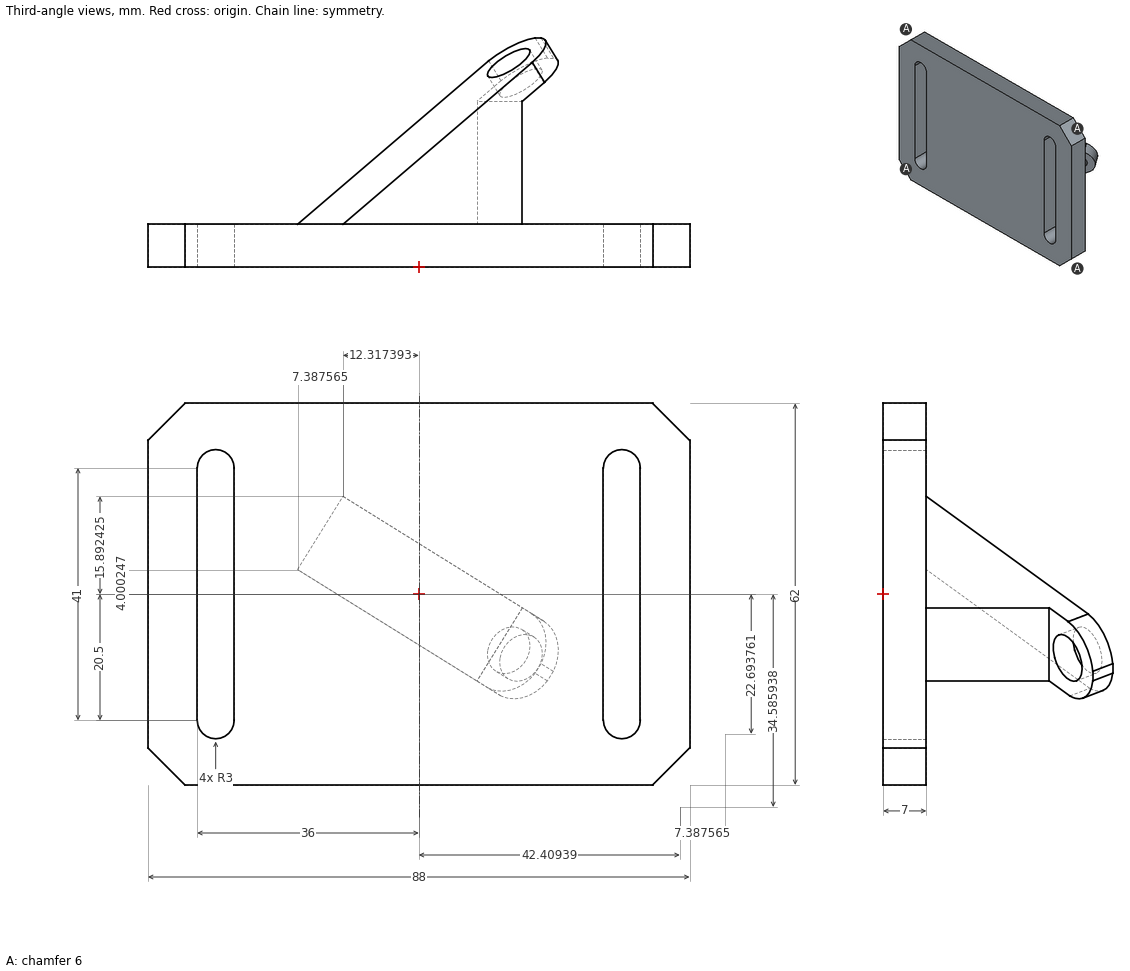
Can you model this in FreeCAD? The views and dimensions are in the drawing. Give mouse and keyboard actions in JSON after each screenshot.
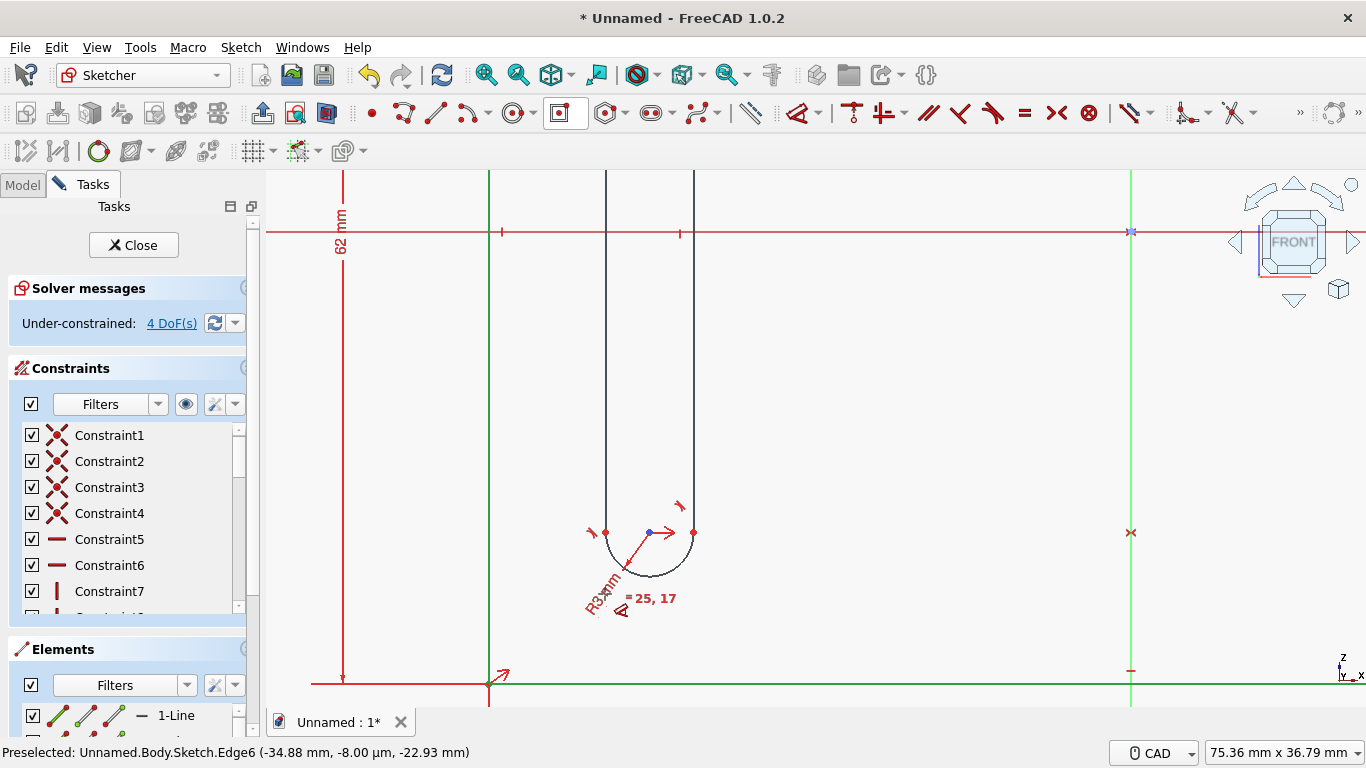
{"action": "left_click", "coordinate": [606, 353]}
{"action": "left_click", "coordinate": [572, 365]}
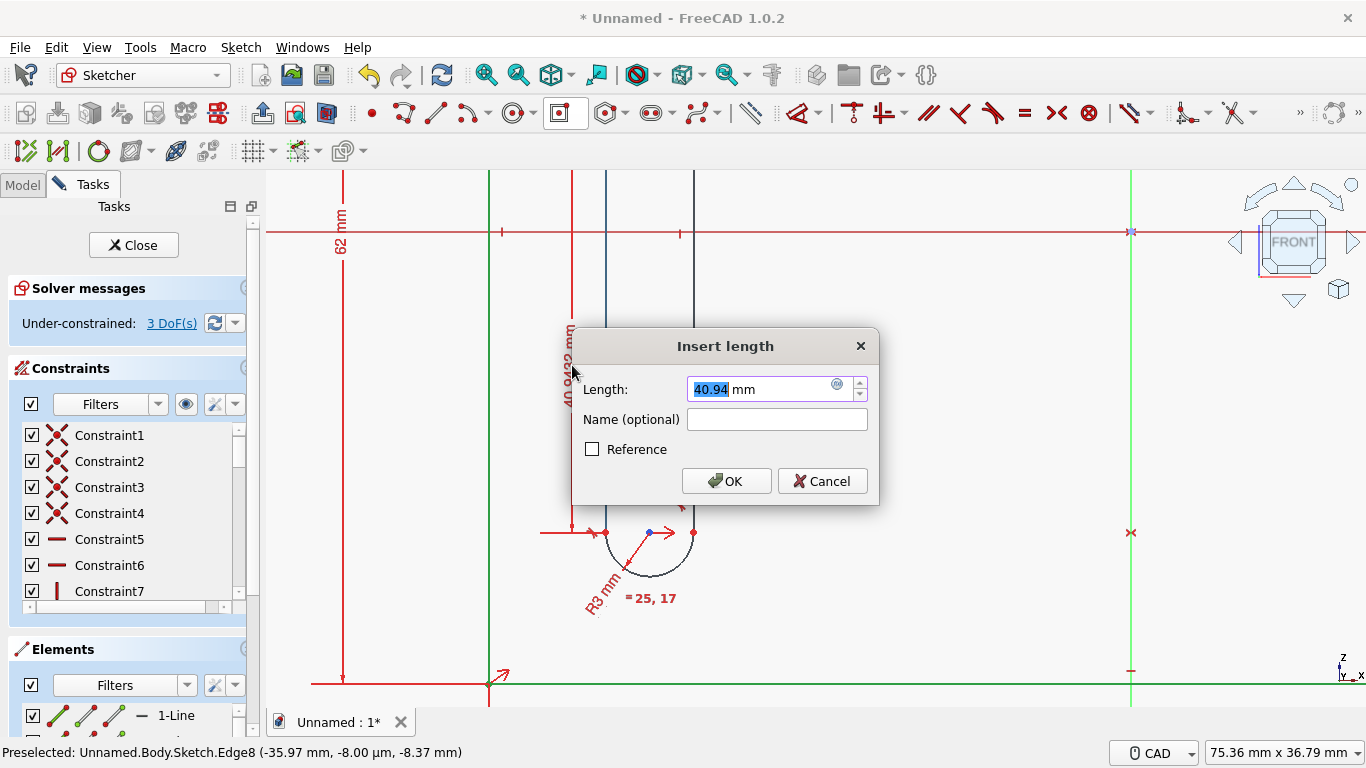
{"action": "type", "text": "41"}
{"action": "key", "text": "Return"}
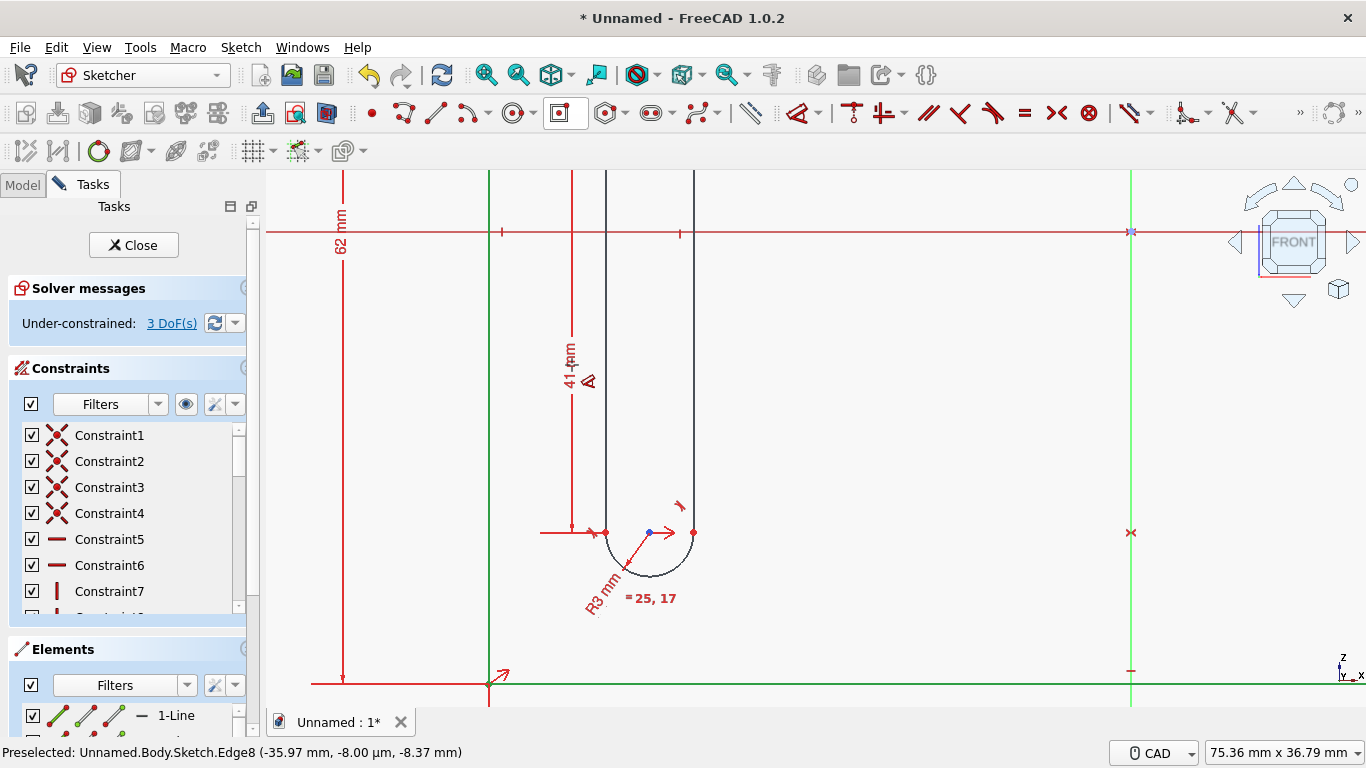
{"action": "scroll", "coordinate": [524, 559], "scroll_direction": "down", "scroll_amount": 5}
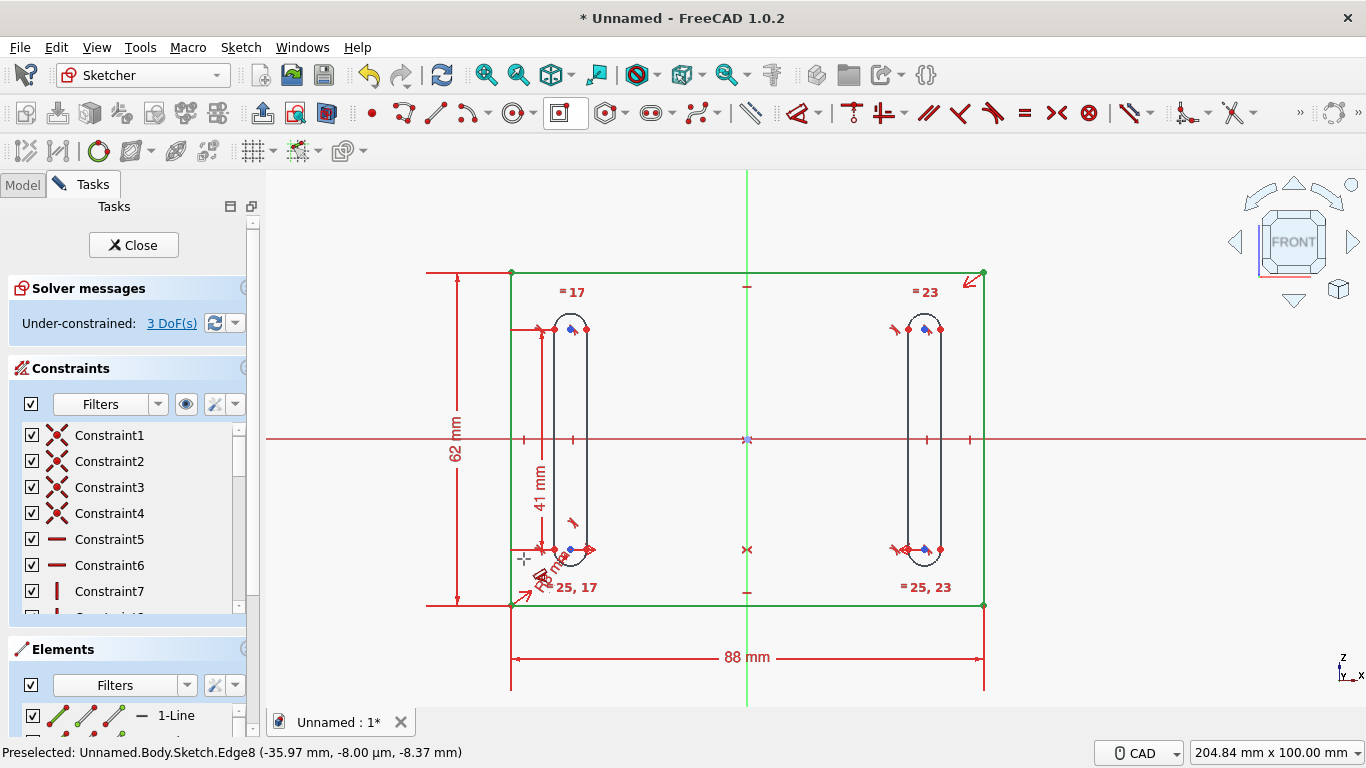
{"action": "left_click", "coordinate": [908, 484]}
{"action": "left_click", "coordinate": [874, 389]}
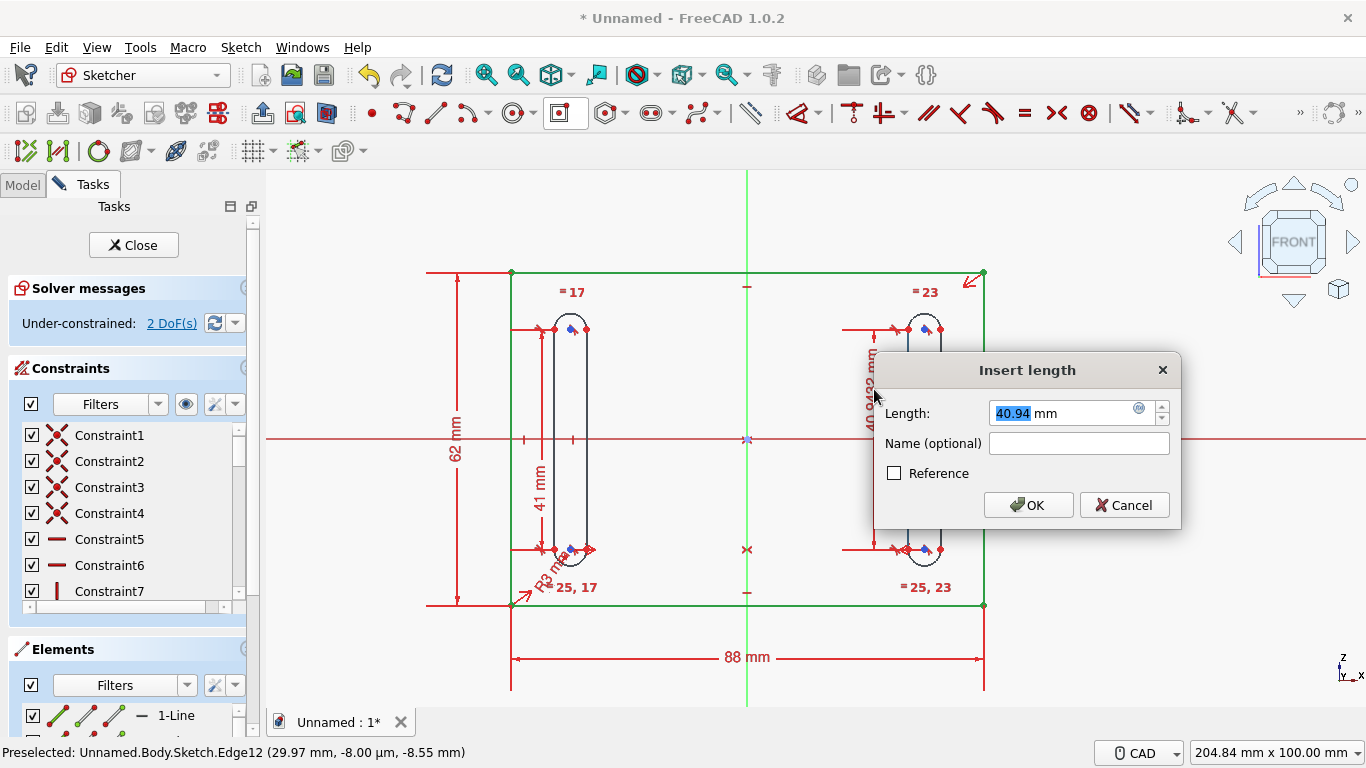
{"action": "type", "text": "41"}
{"action": "key", "text": "Return"}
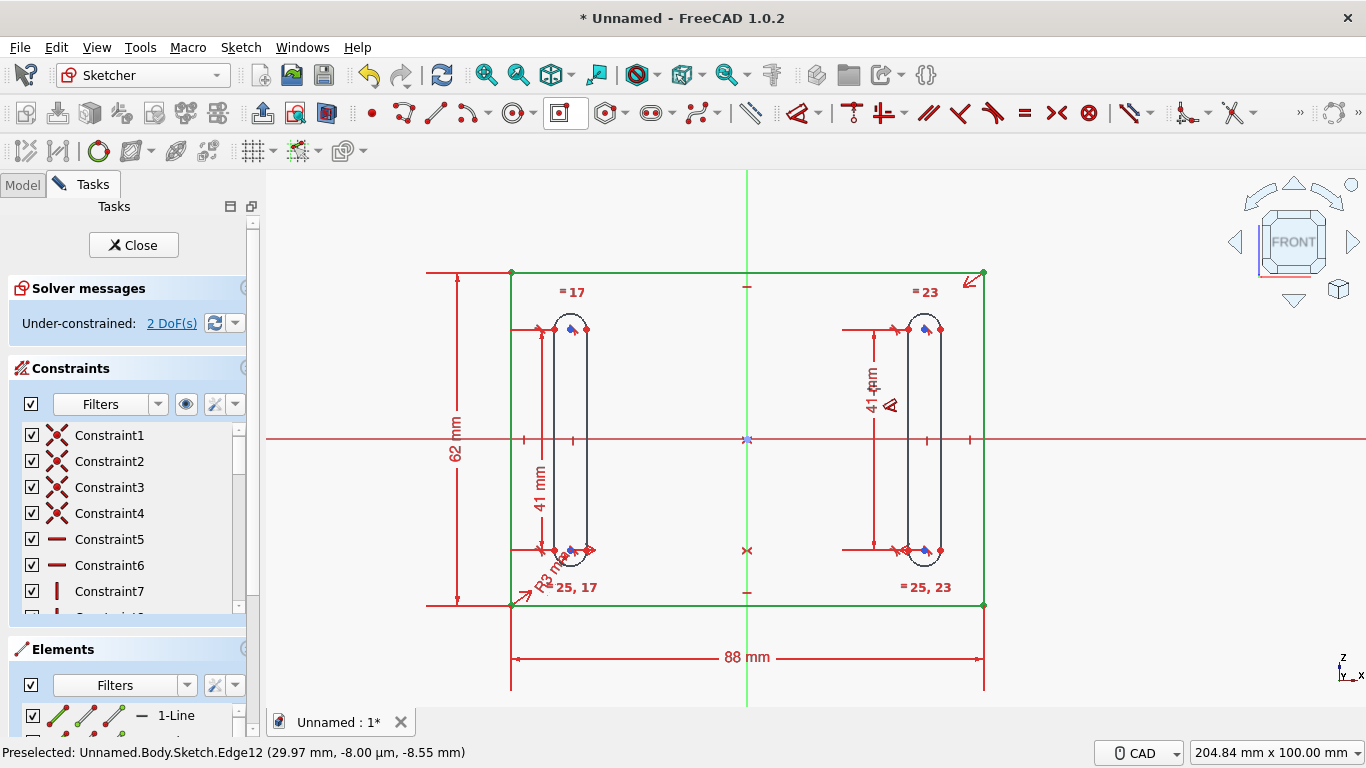
{"action": "left_click", "coordinate": [554, 550]}
{"action": "left_click", "coordinate": [651, 584]}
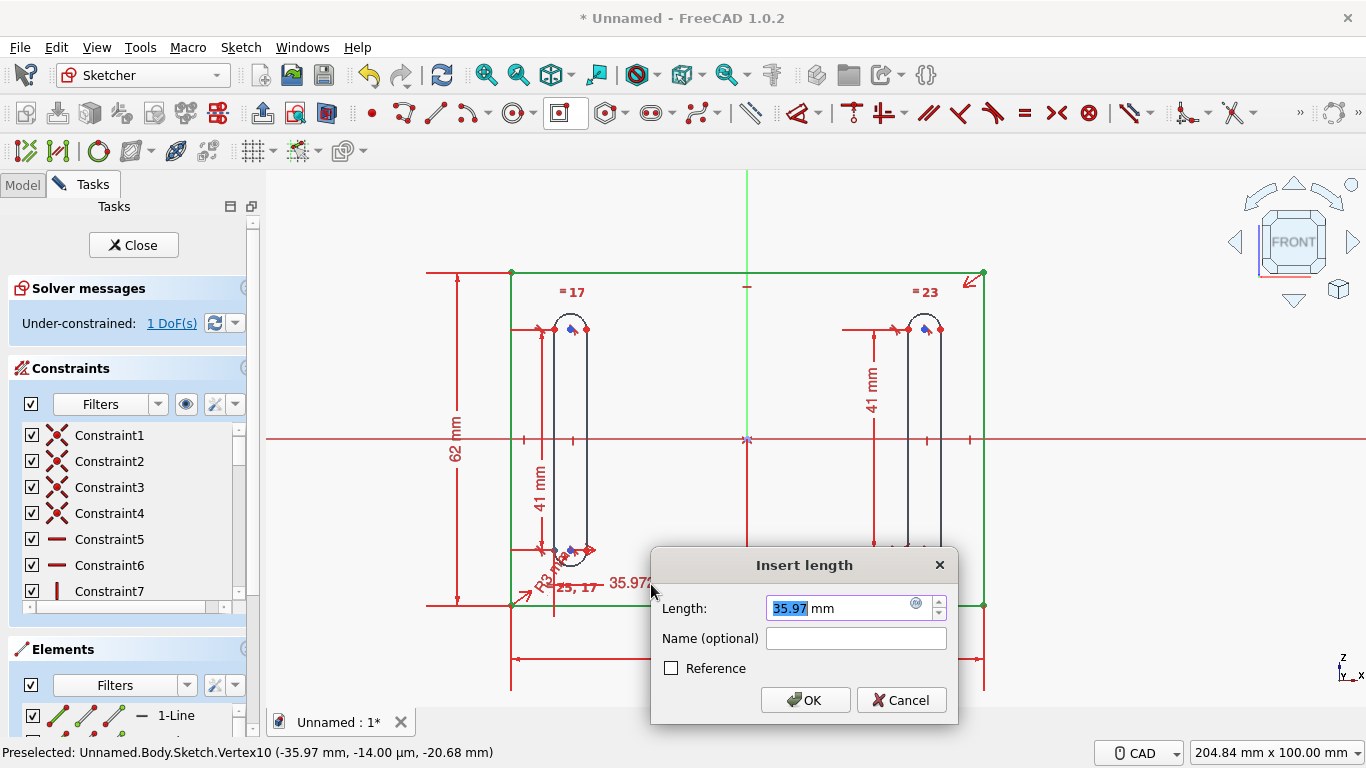
{"action": "type", "text": "36"}
{"action": "key", "text": "Return"}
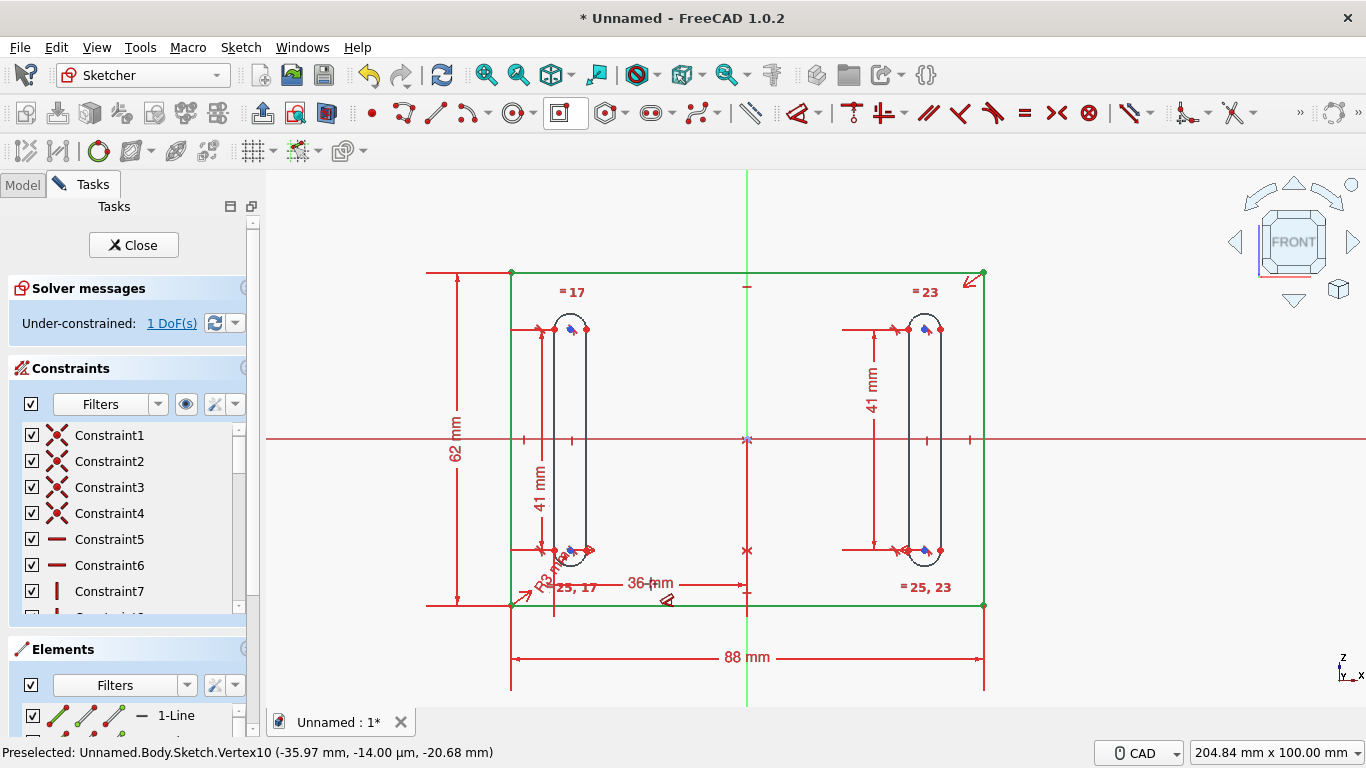
{"action": "left_click", "coordinate": [554, 550]}
{"action": "left_click", "coordinate": [781, 495]}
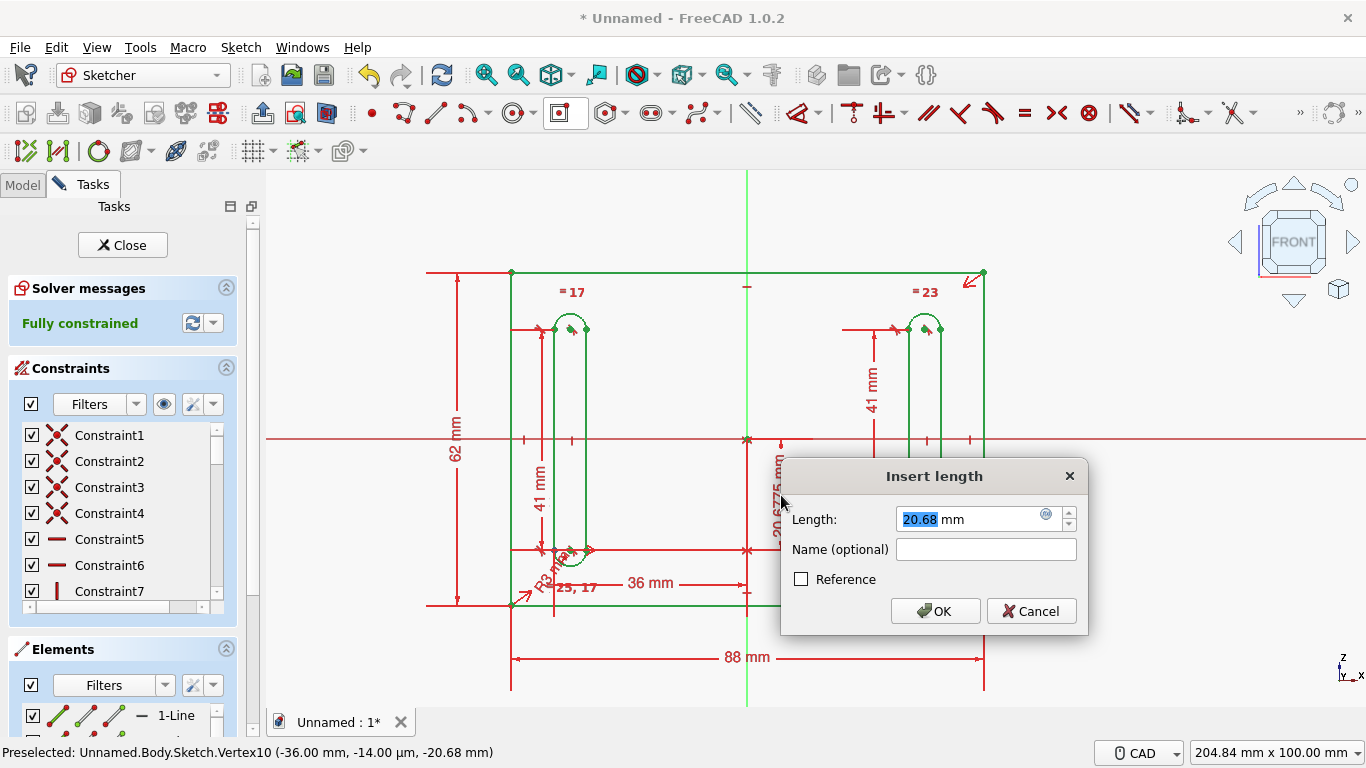
{"action": "type", "text": "20.5"}
{"action": "key", "text": "Return"}
{"action": "key", "text": "Escape"}